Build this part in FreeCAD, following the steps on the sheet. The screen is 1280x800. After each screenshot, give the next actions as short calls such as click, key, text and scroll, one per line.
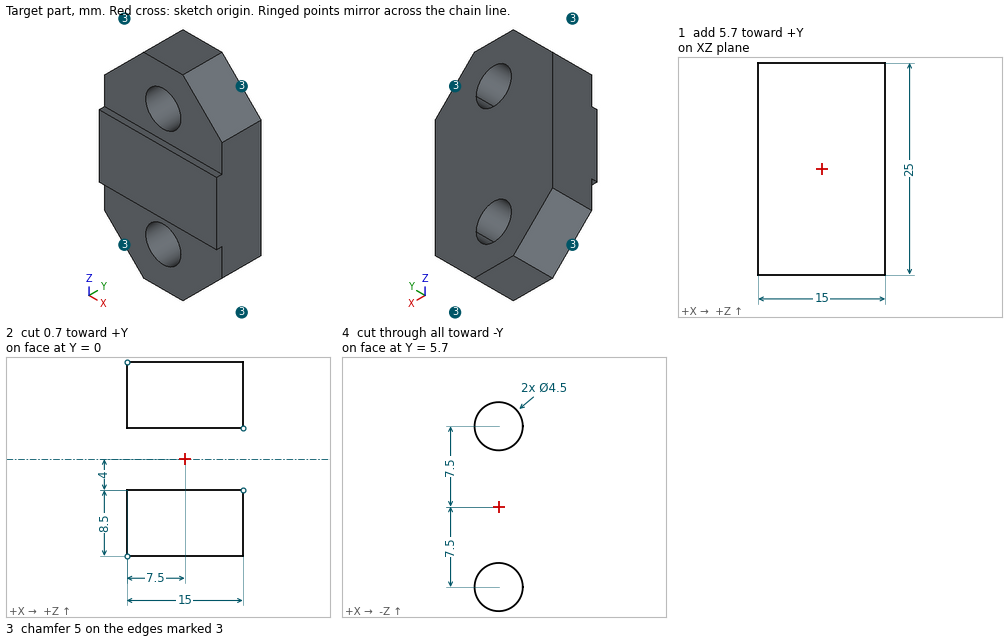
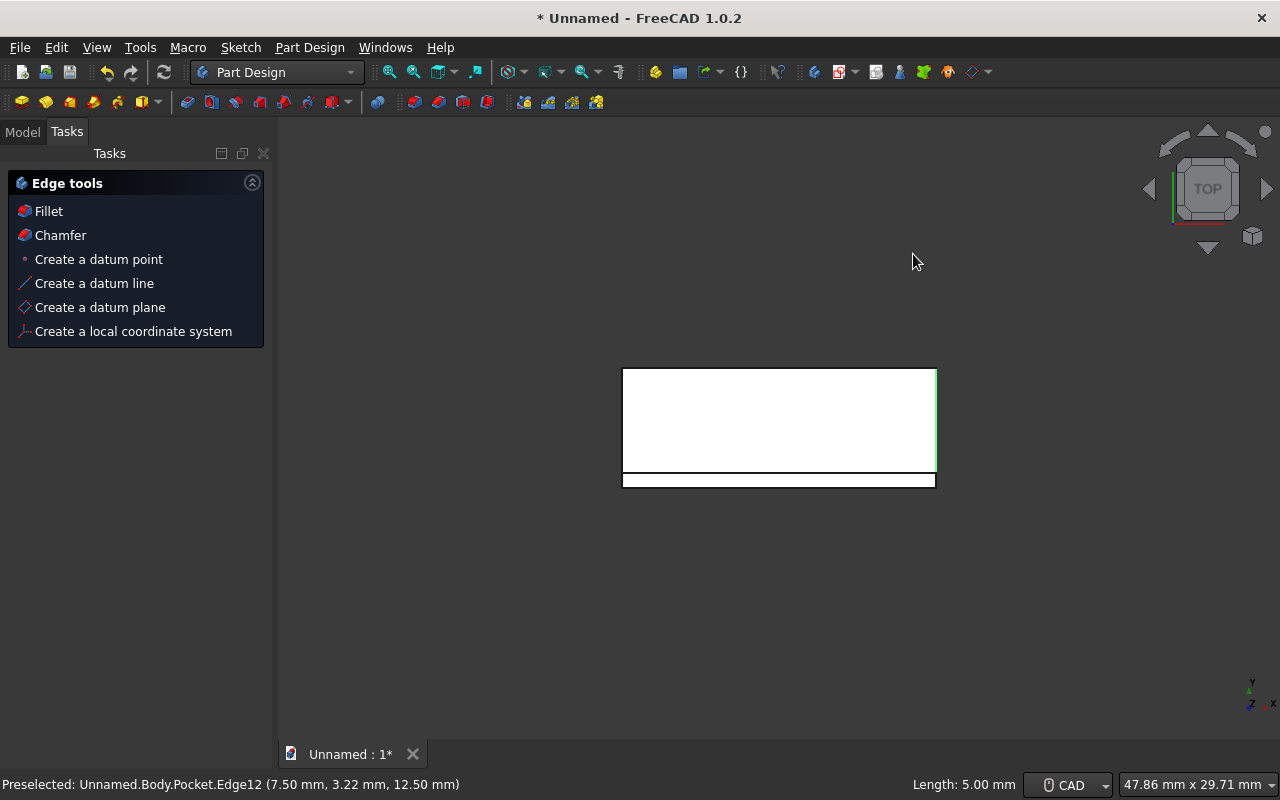
click(622, 420, ctrl)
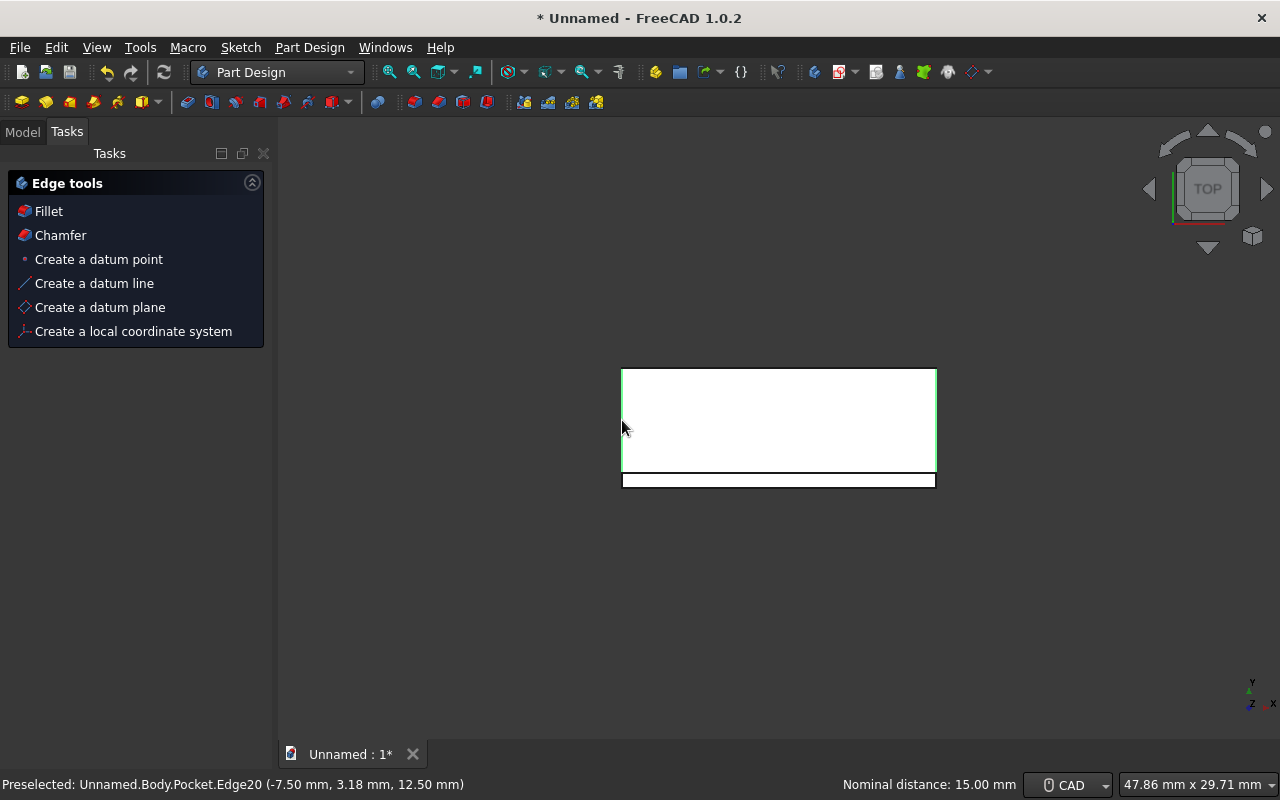
key(1)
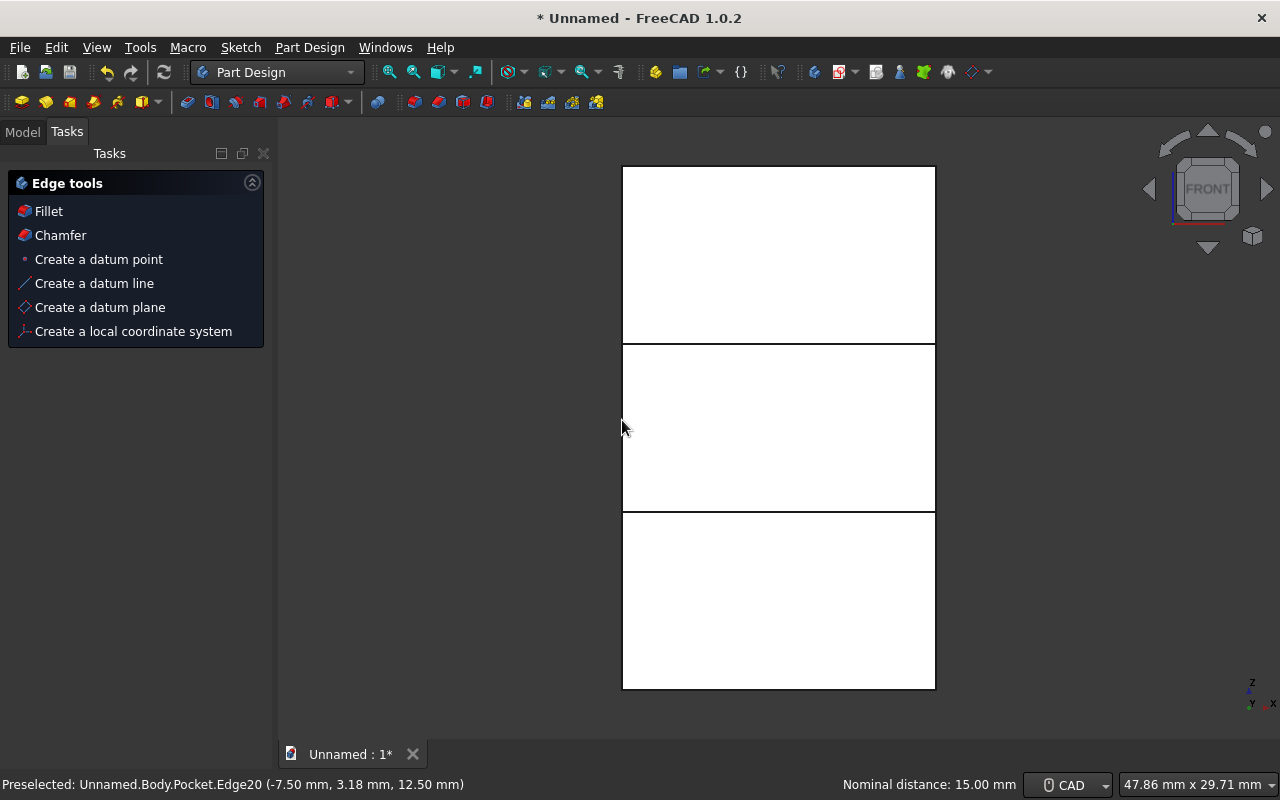
key(3)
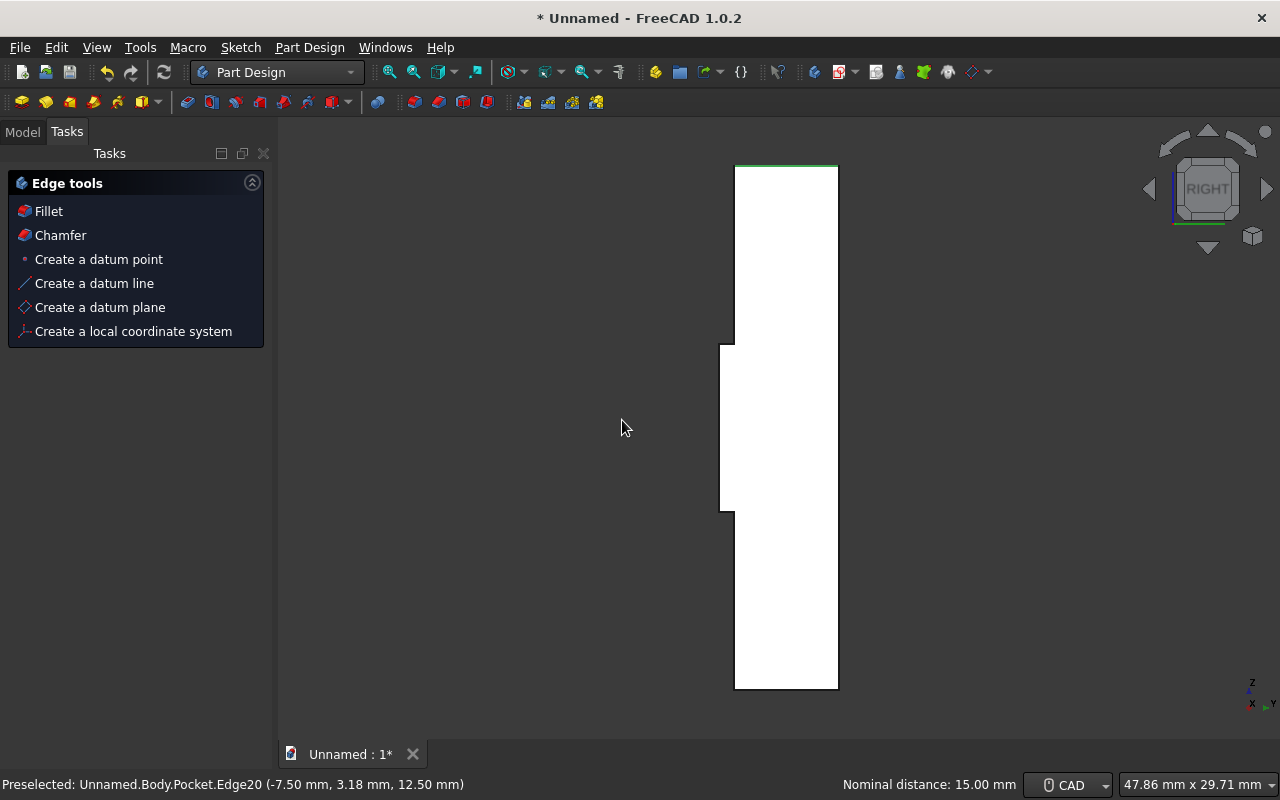
click(786, 689, ctrl)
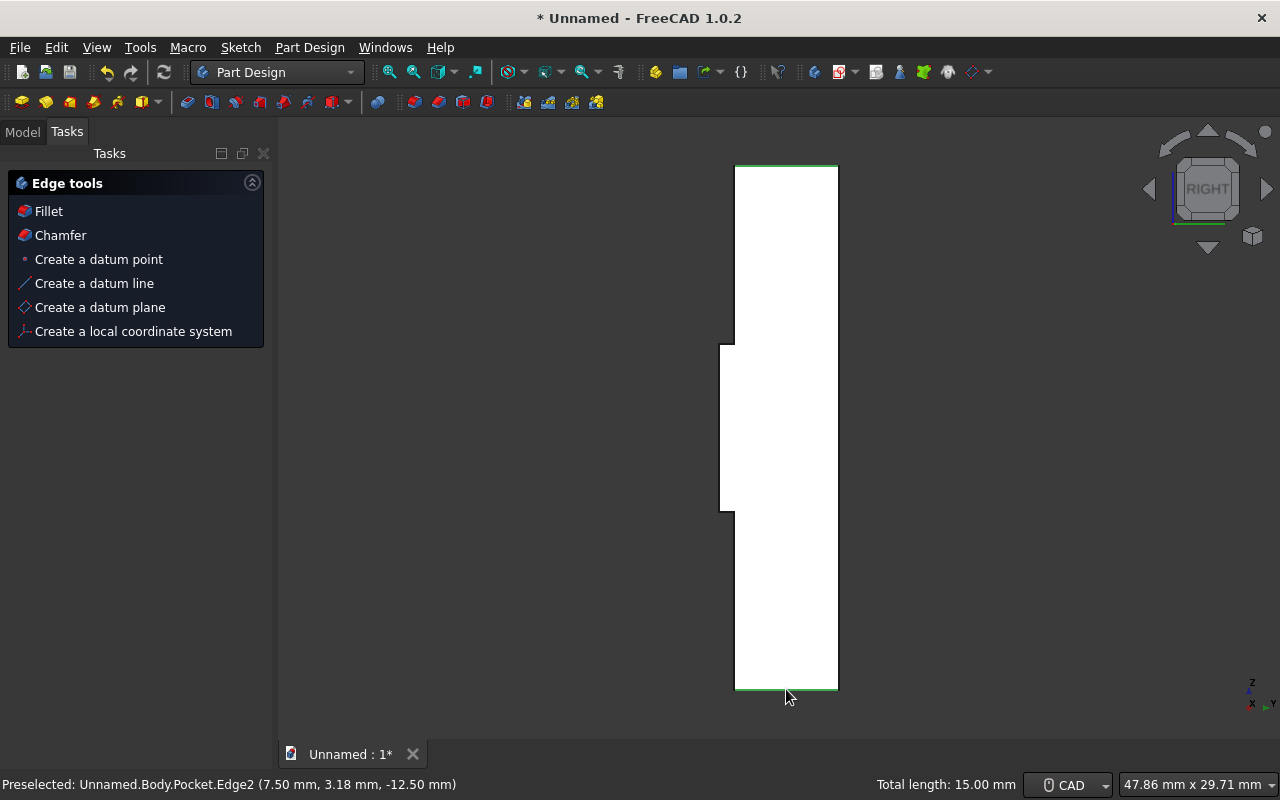
key(5)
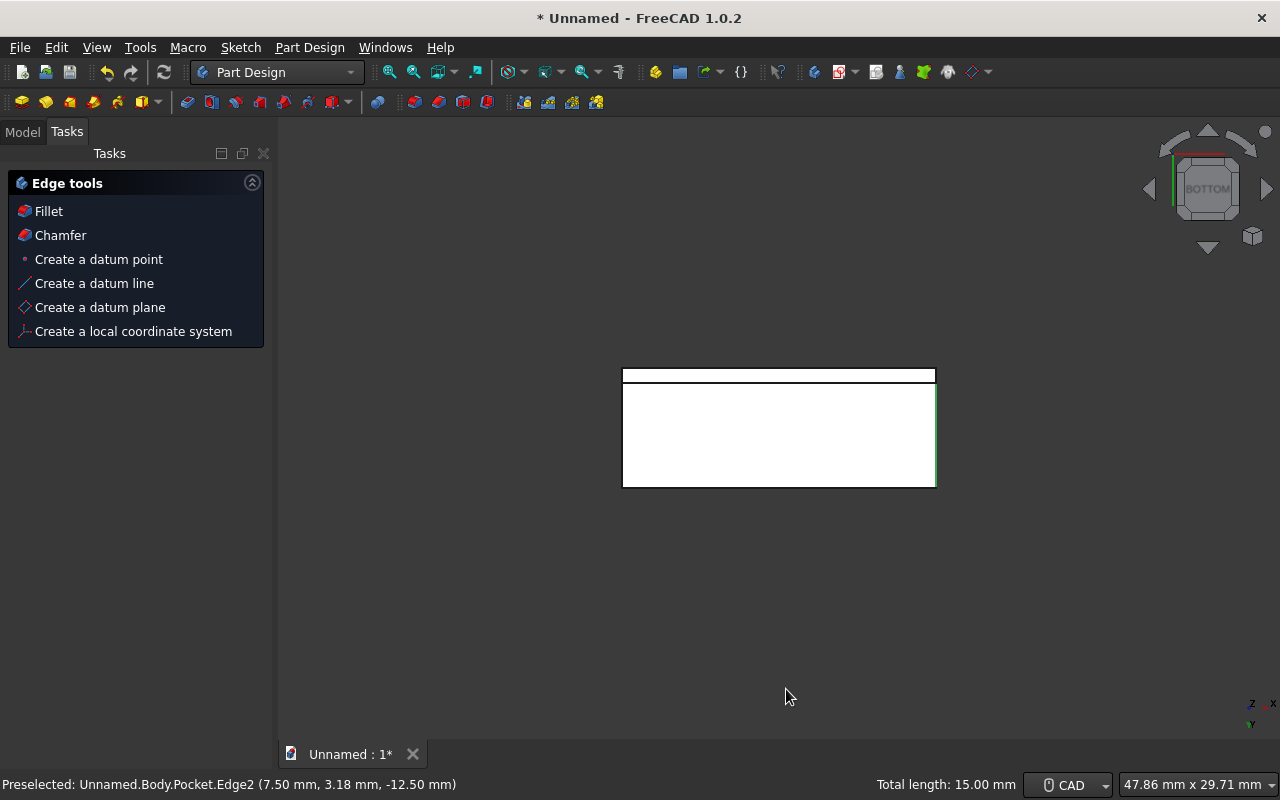
key(v)
key(f)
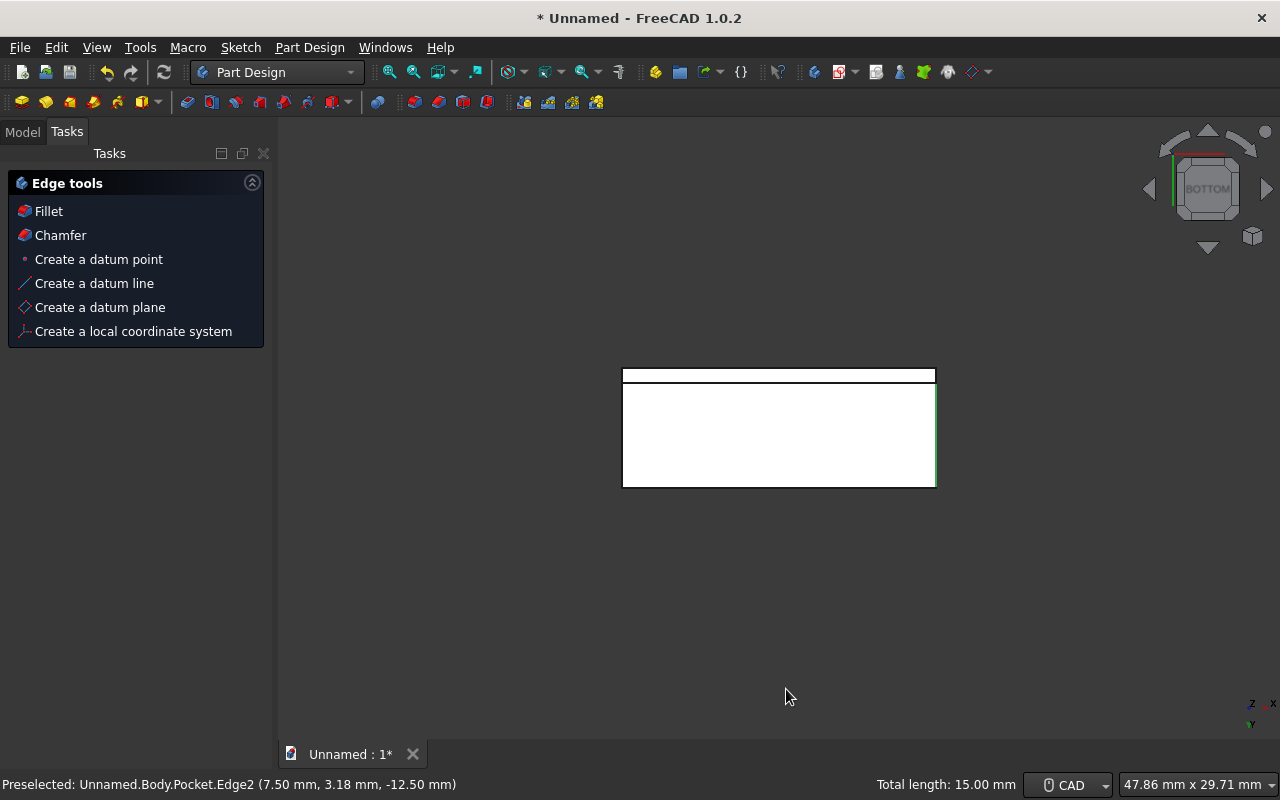
click(622, 434, ctrl)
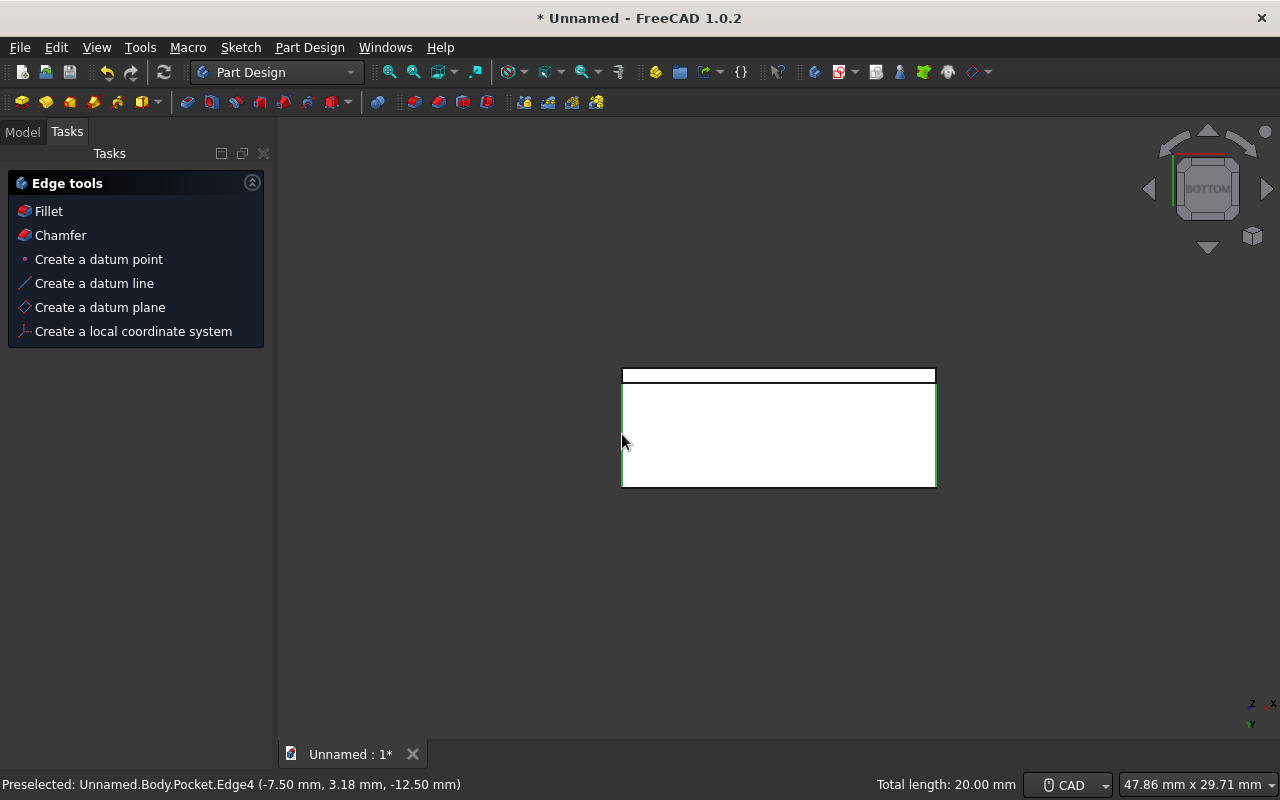
click(440, 102)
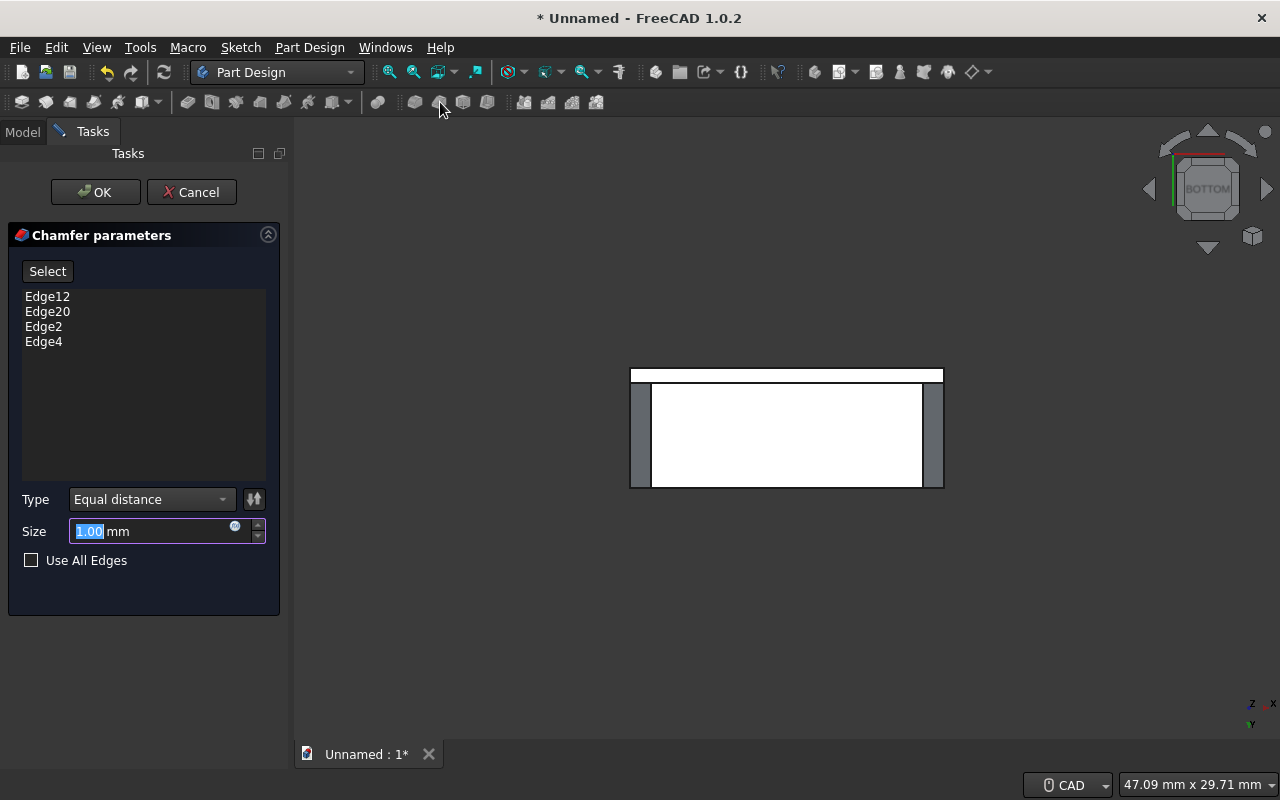
text(5)
key(Tab)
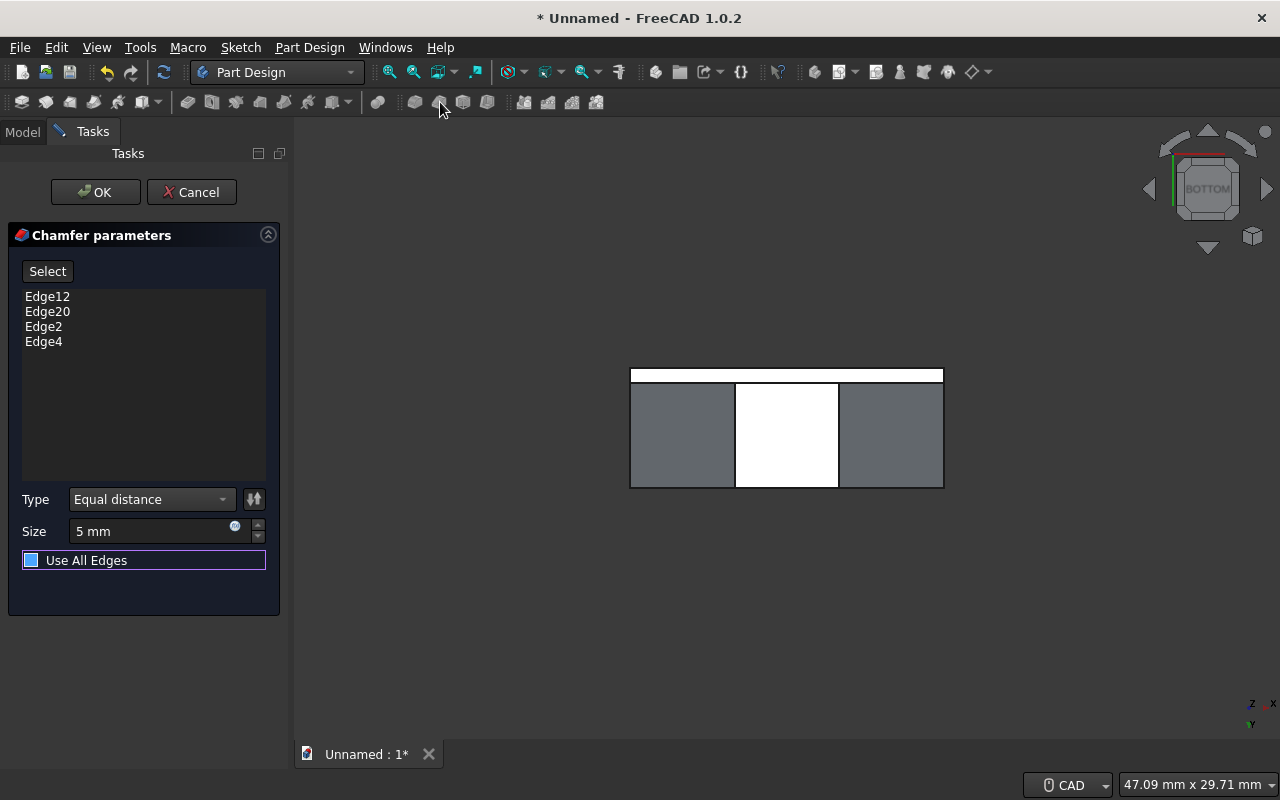
click(96, 192)